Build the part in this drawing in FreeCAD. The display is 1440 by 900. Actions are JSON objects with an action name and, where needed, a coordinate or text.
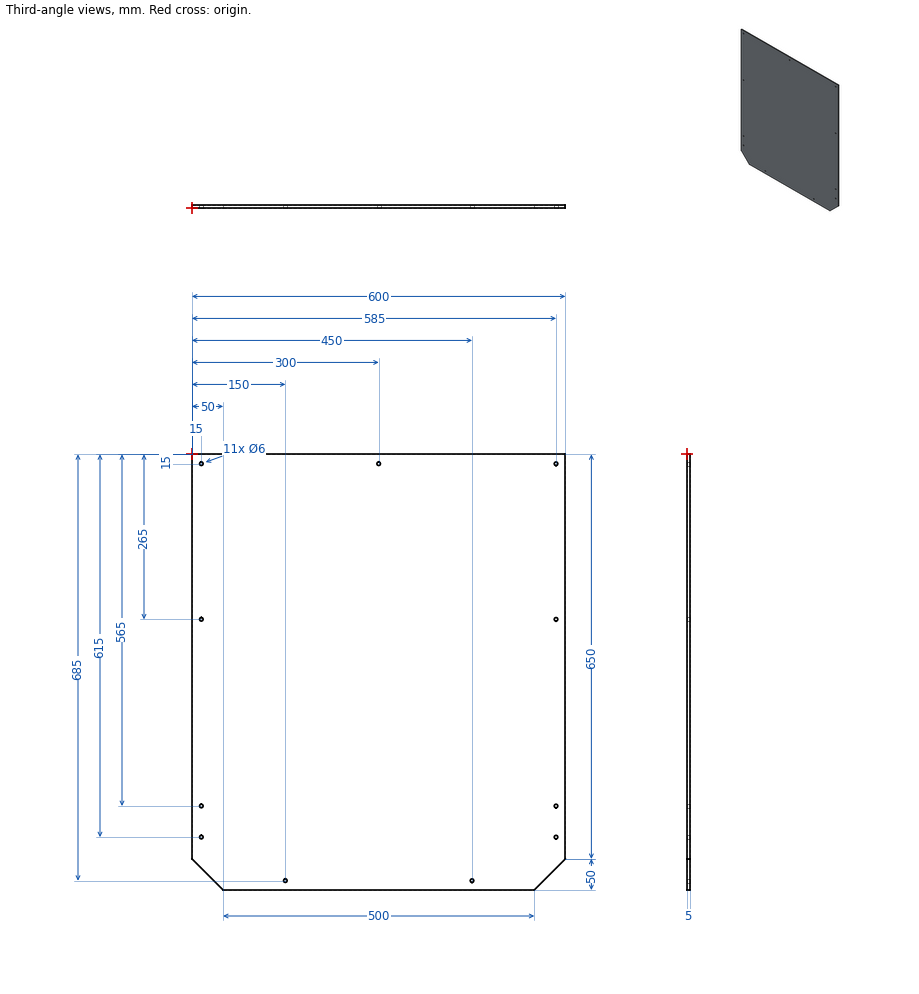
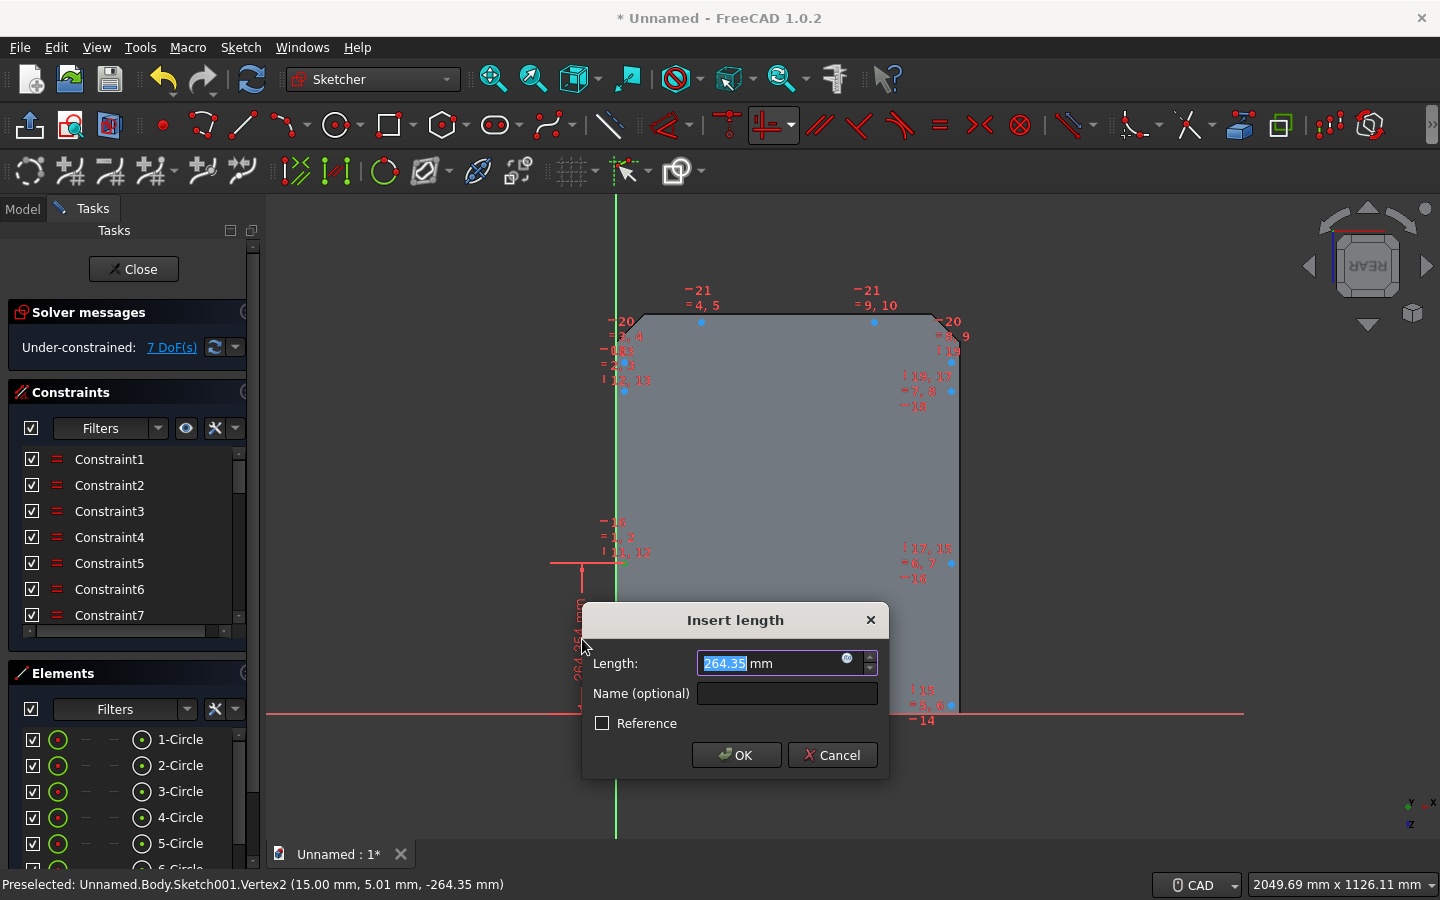
{"action": "type", "text": "265"}
{"action": "key", "text": "Return"}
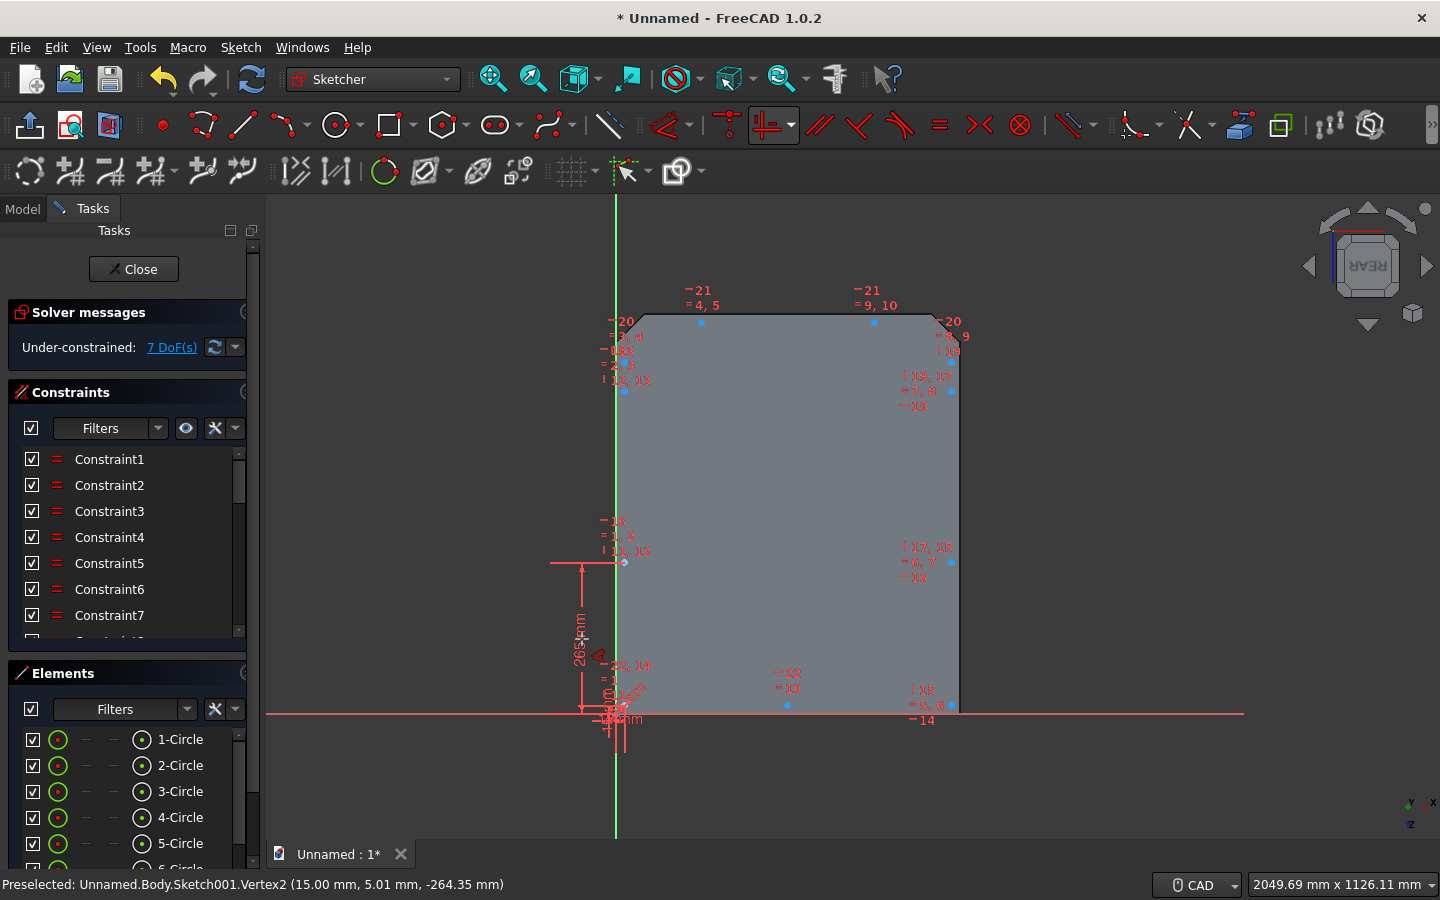
{"action": "left_click", "coordinate": [625, 391]}
{"action": "left_click", "coordinate": [582, 553]}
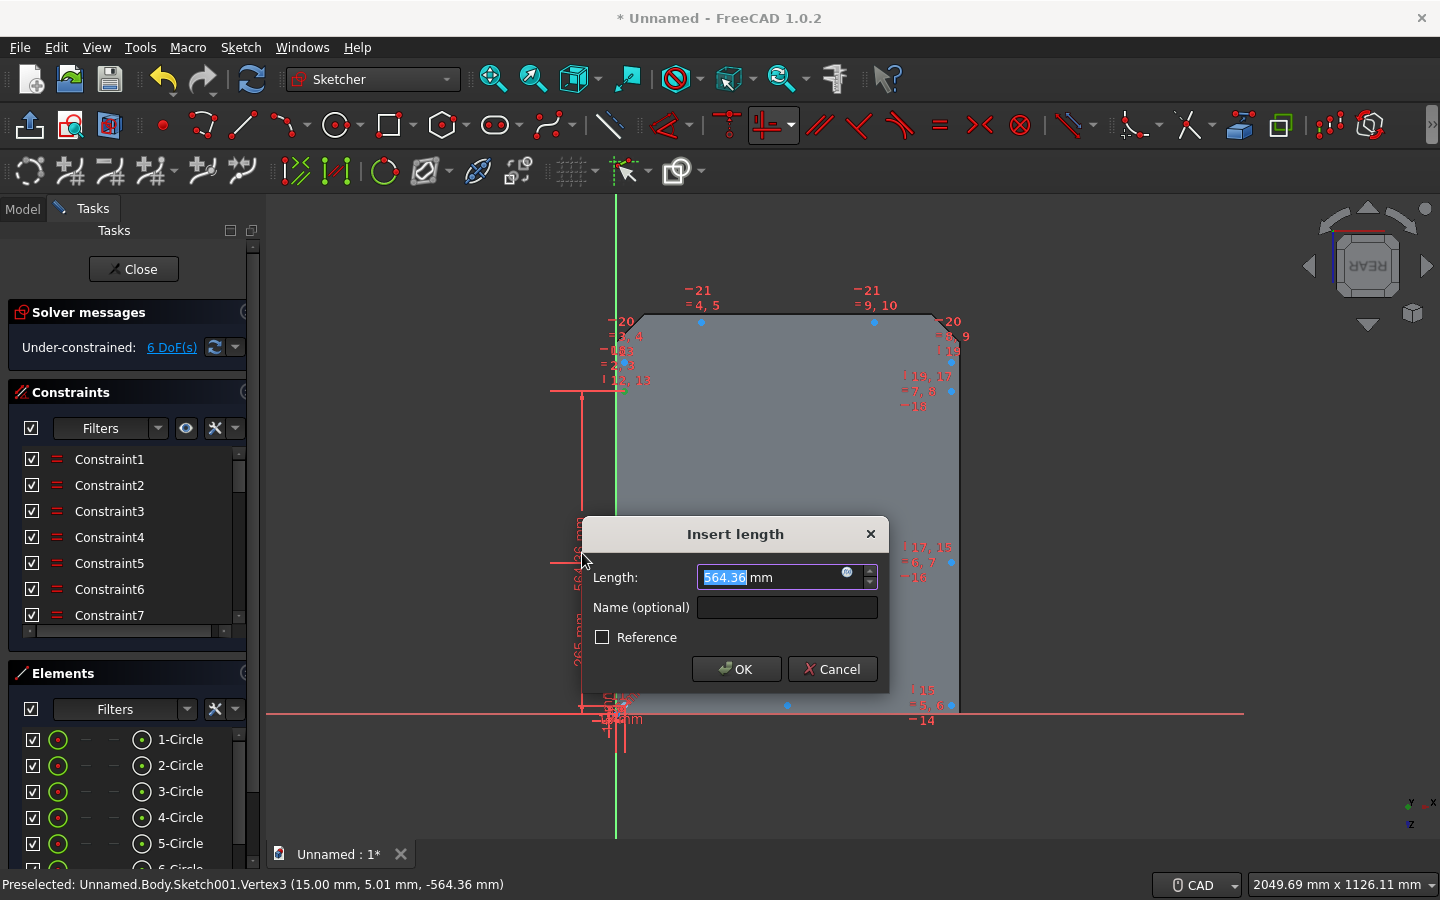
{"action": "type", "text": "565"}
{"action": "key", "text": "Return"}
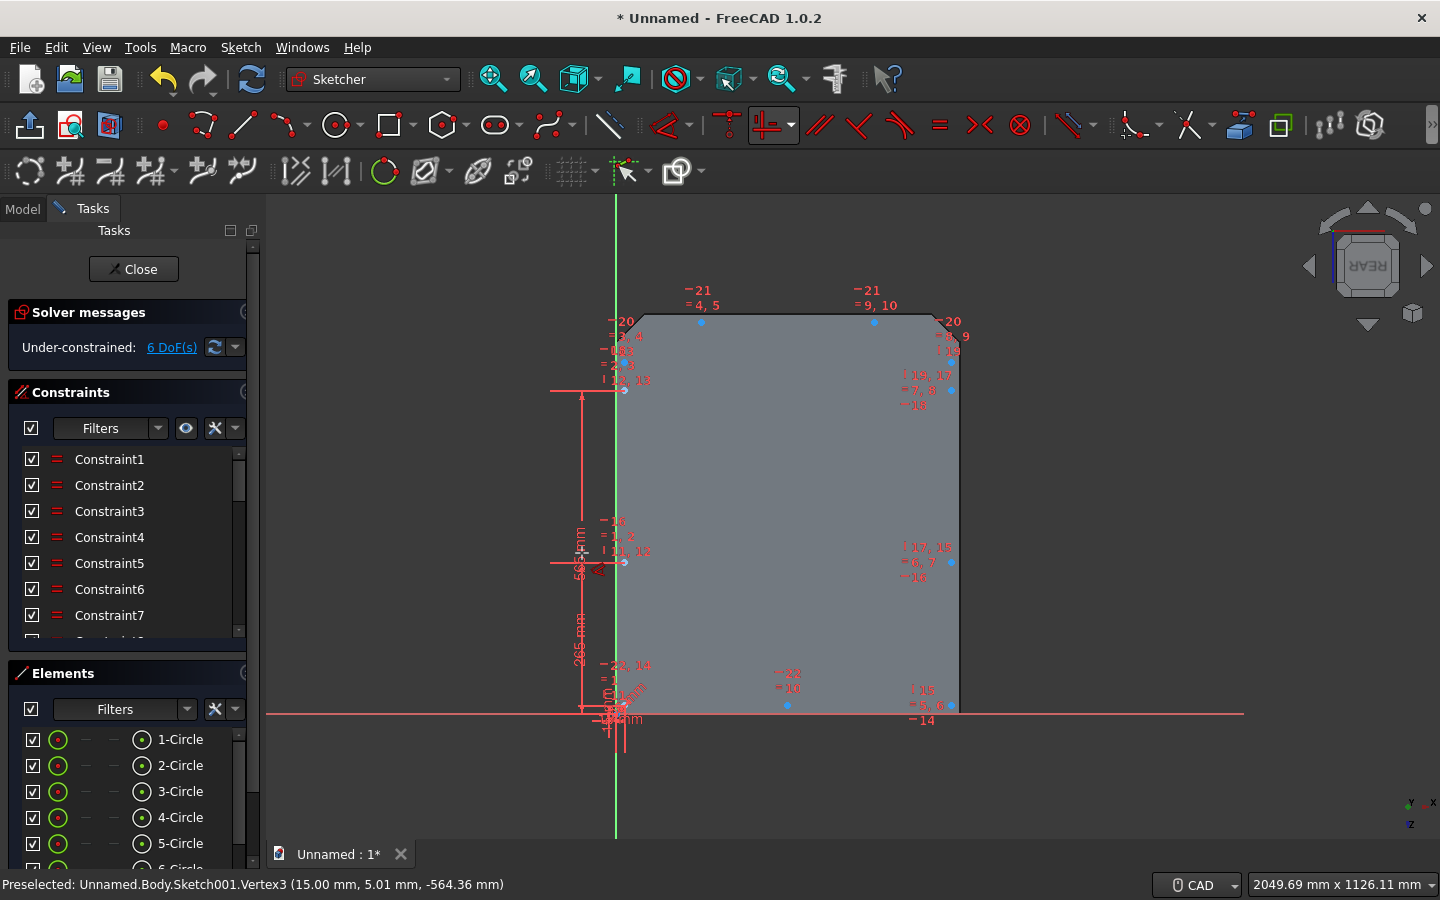
{"action": "left_click", "coordinate": [625, 363]}
{"action": "left_click", "coordinate": [582, 458]}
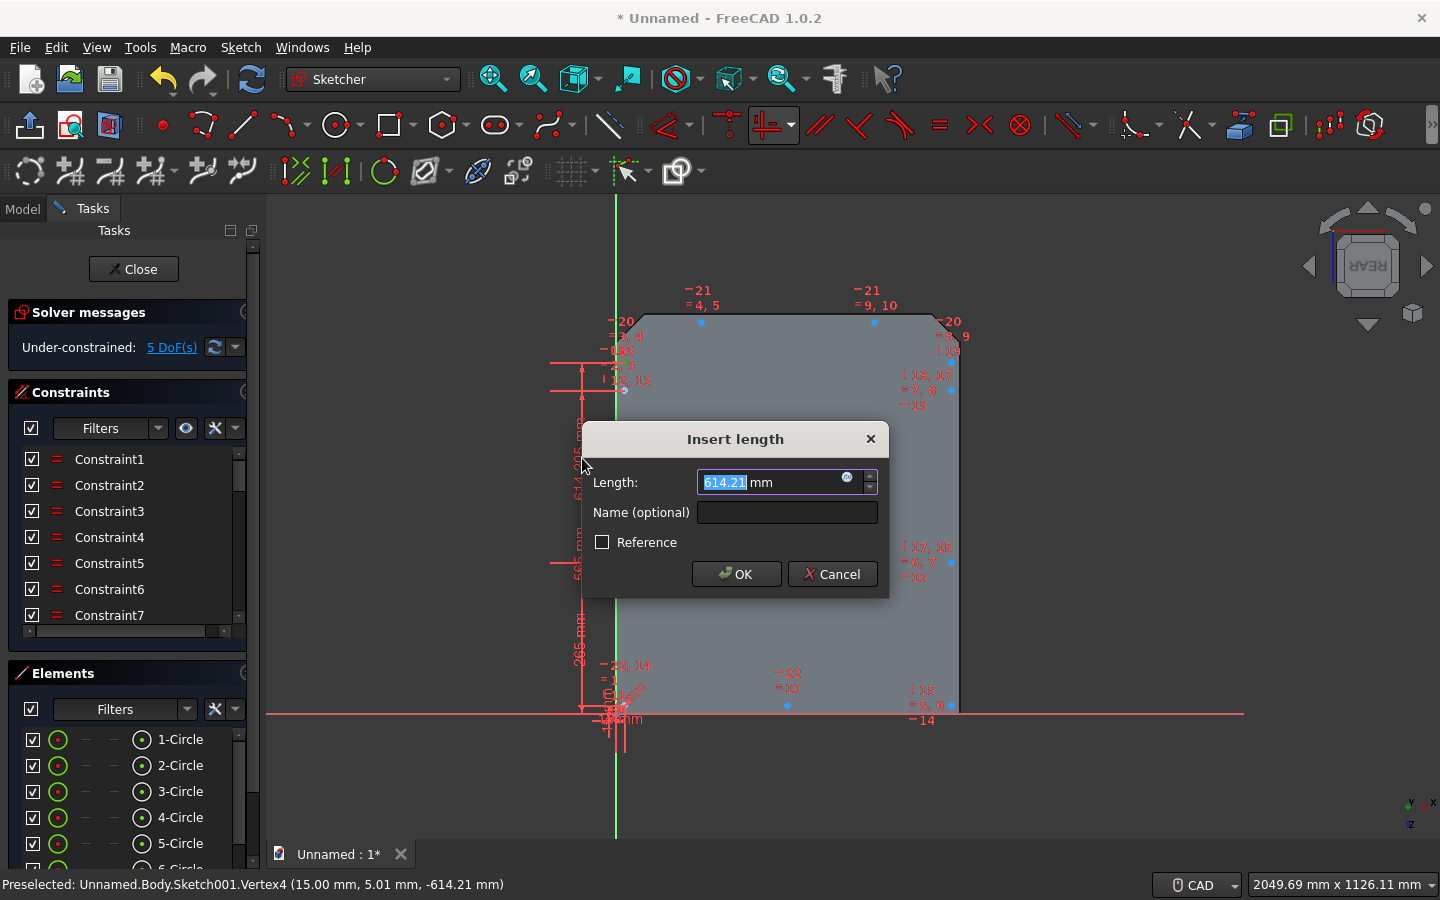
{"action": "type", "text": "615"}
{"action": "key", "text": "Return"}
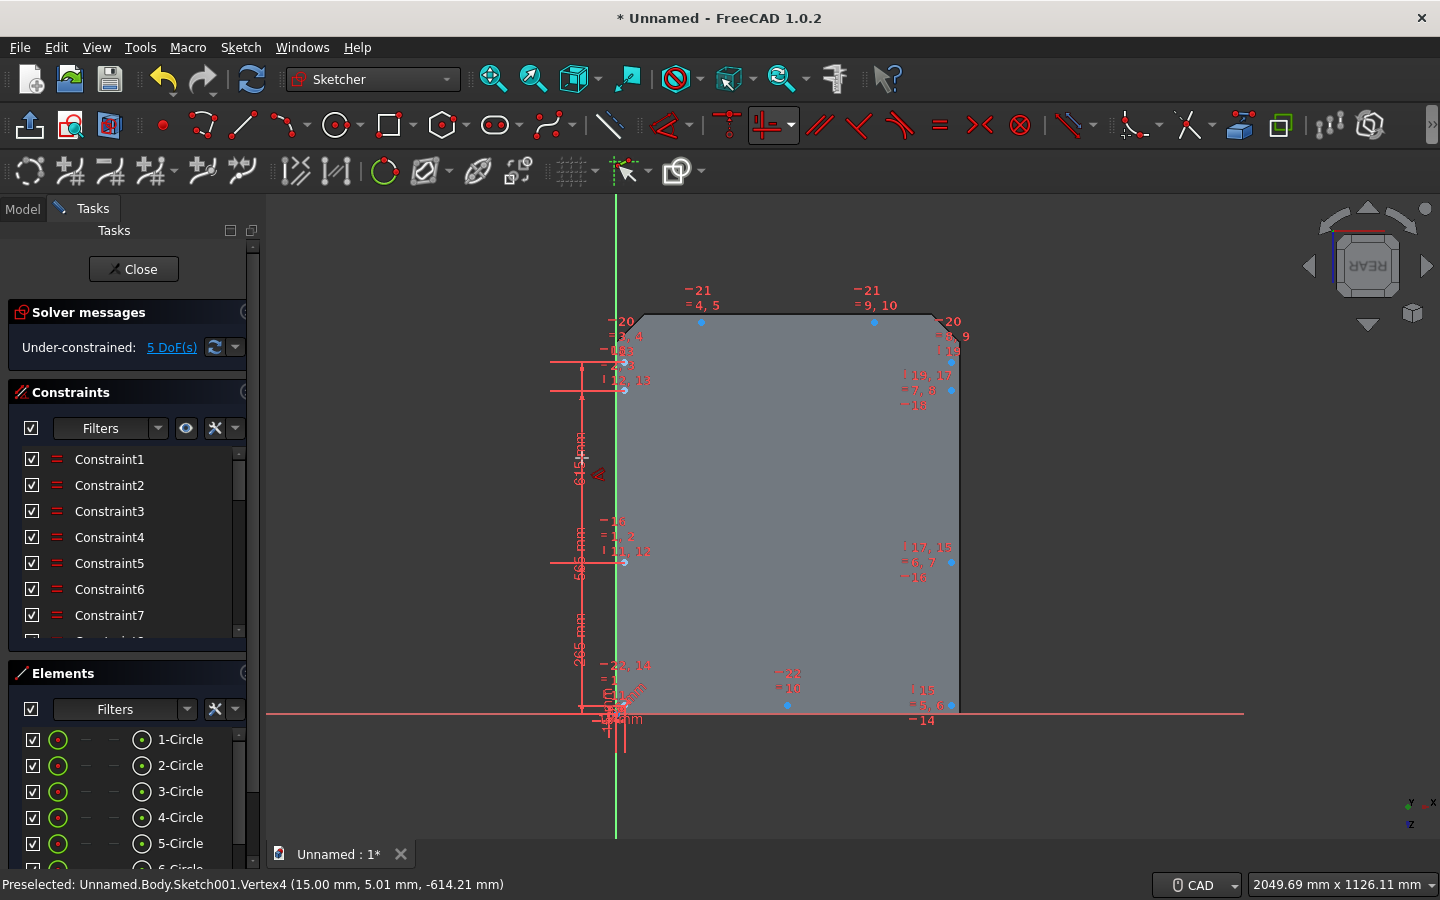
{"action": "left_click", "coordinate": [702, 323]}
{"action": "left_click", "coordinate": [659, 748]}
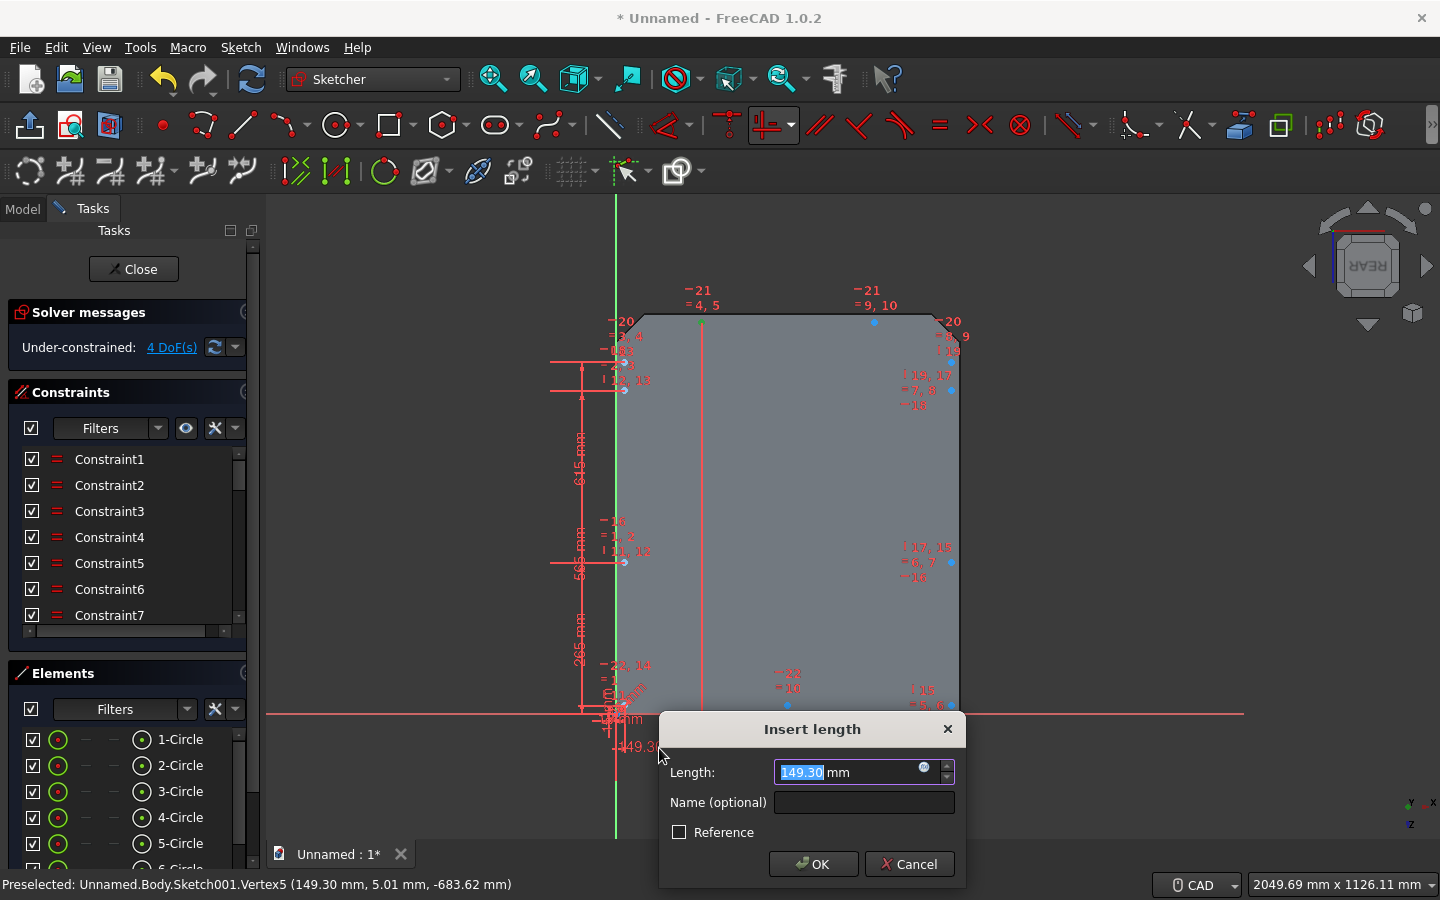
{"action": "type", "text": "150"}
{"action": "key", "text": "Return"}